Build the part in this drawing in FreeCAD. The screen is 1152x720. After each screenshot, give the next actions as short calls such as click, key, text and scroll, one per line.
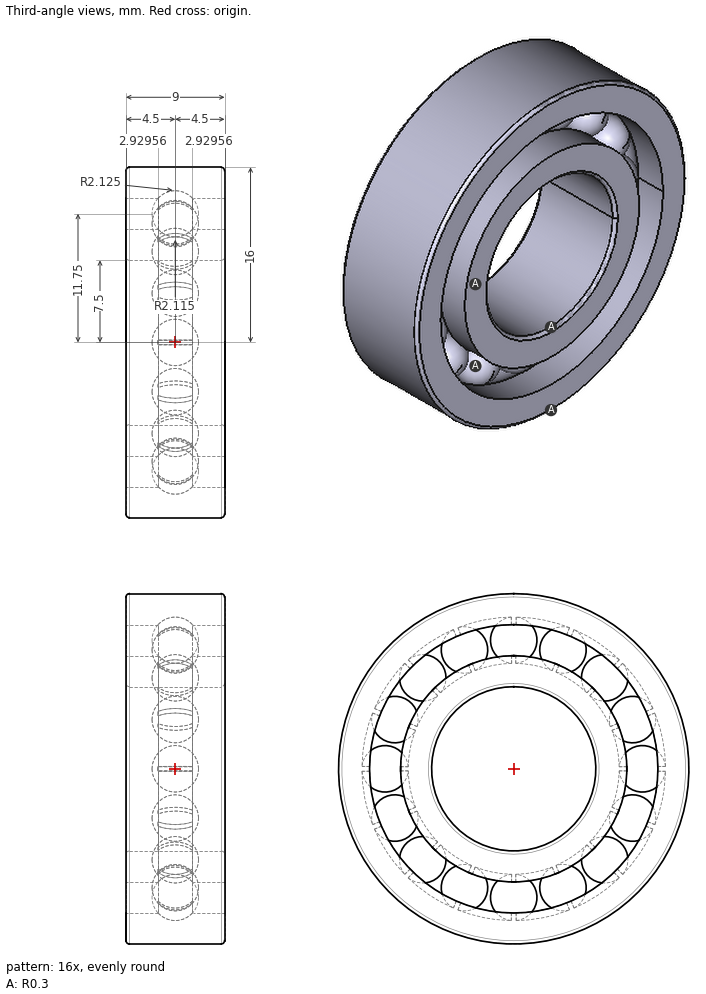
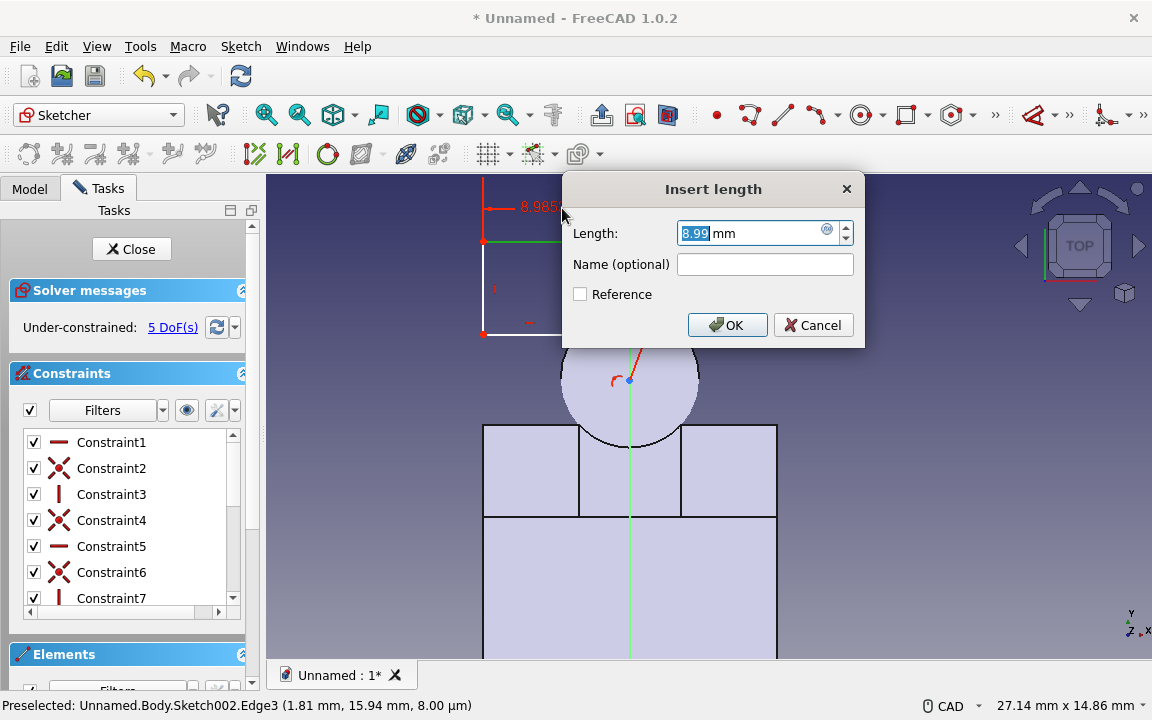
text(9)
key(Return)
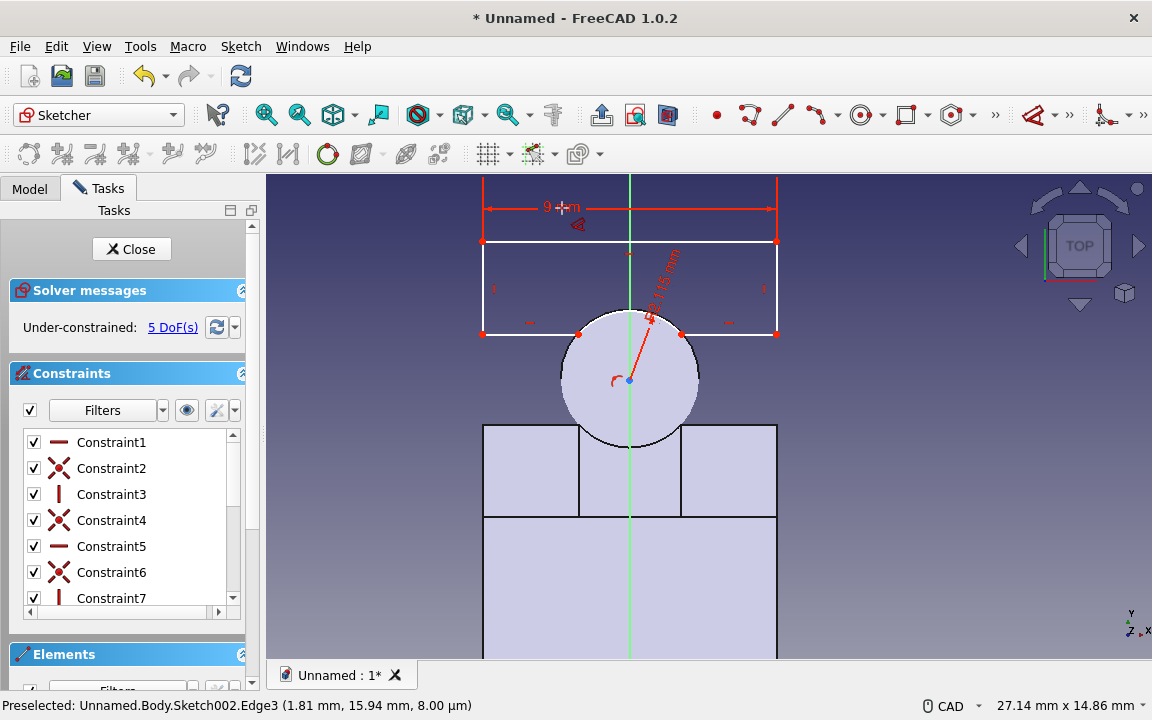
click(777, 242)
click(811, 436)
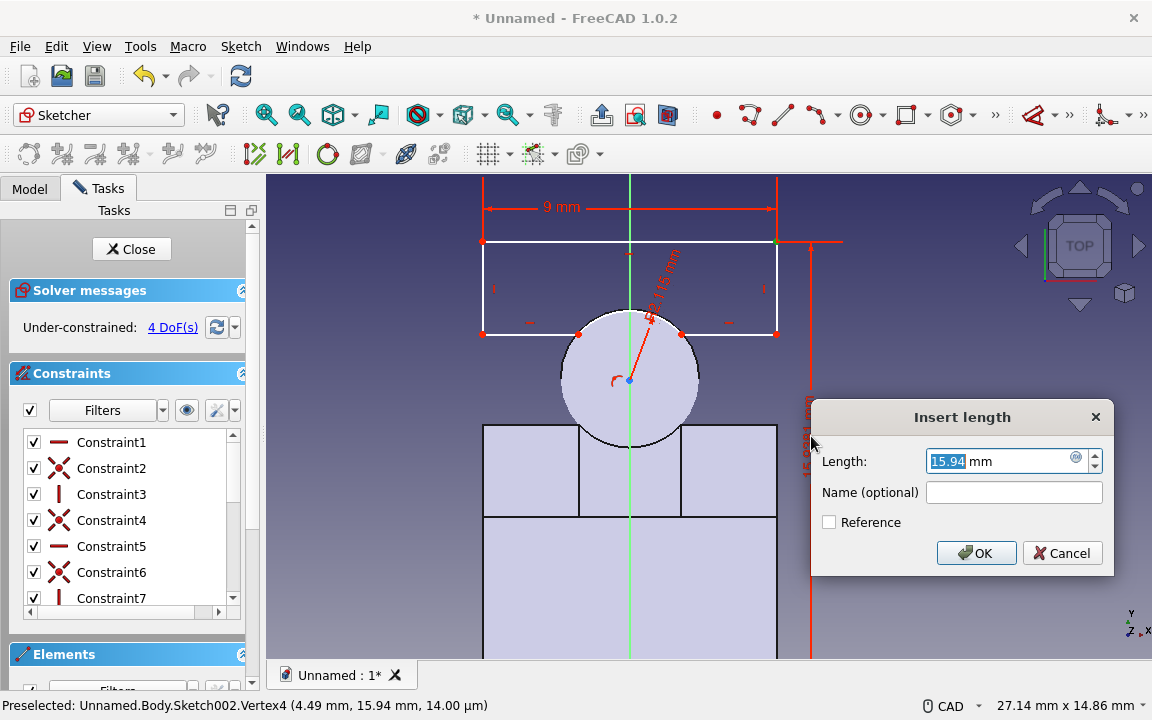
text(16)
key(Return)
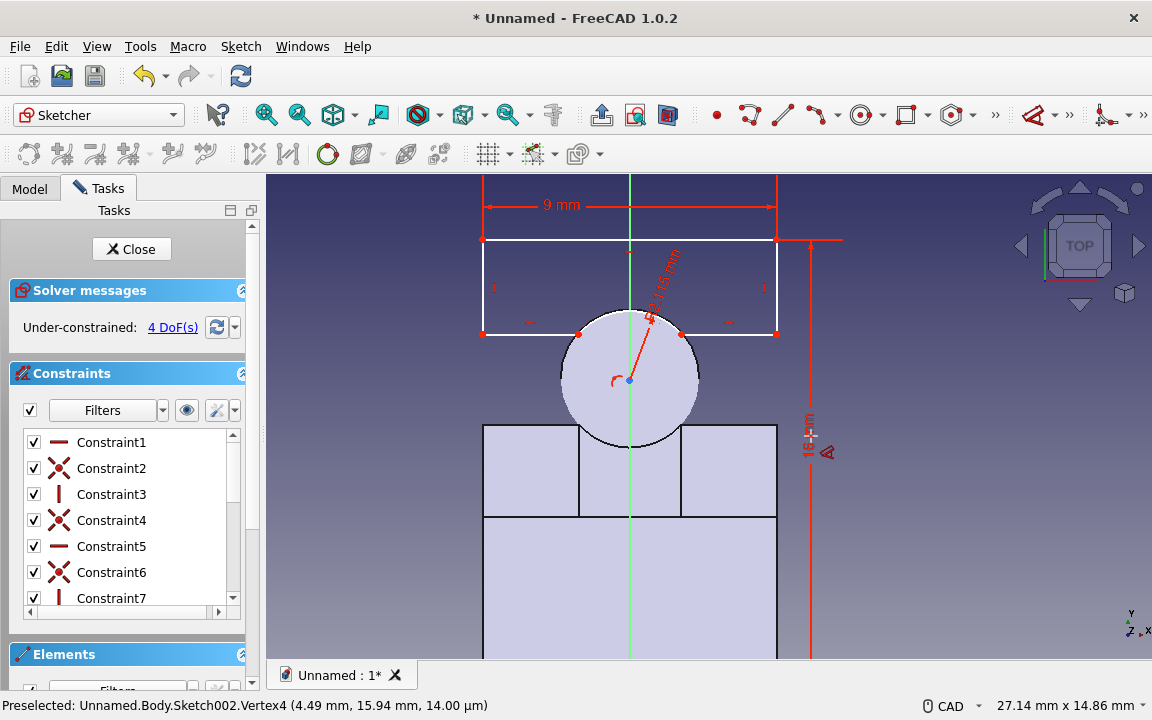
click(777, 335)
click(737, 301)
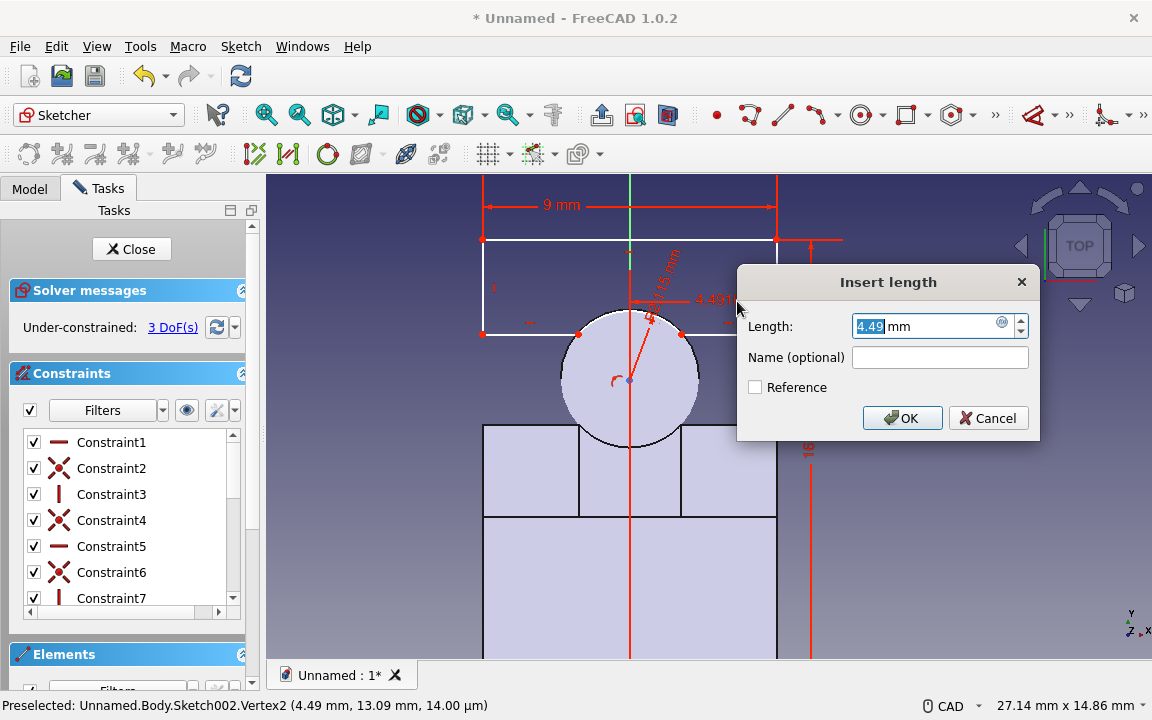
text(4.5)
key(Return)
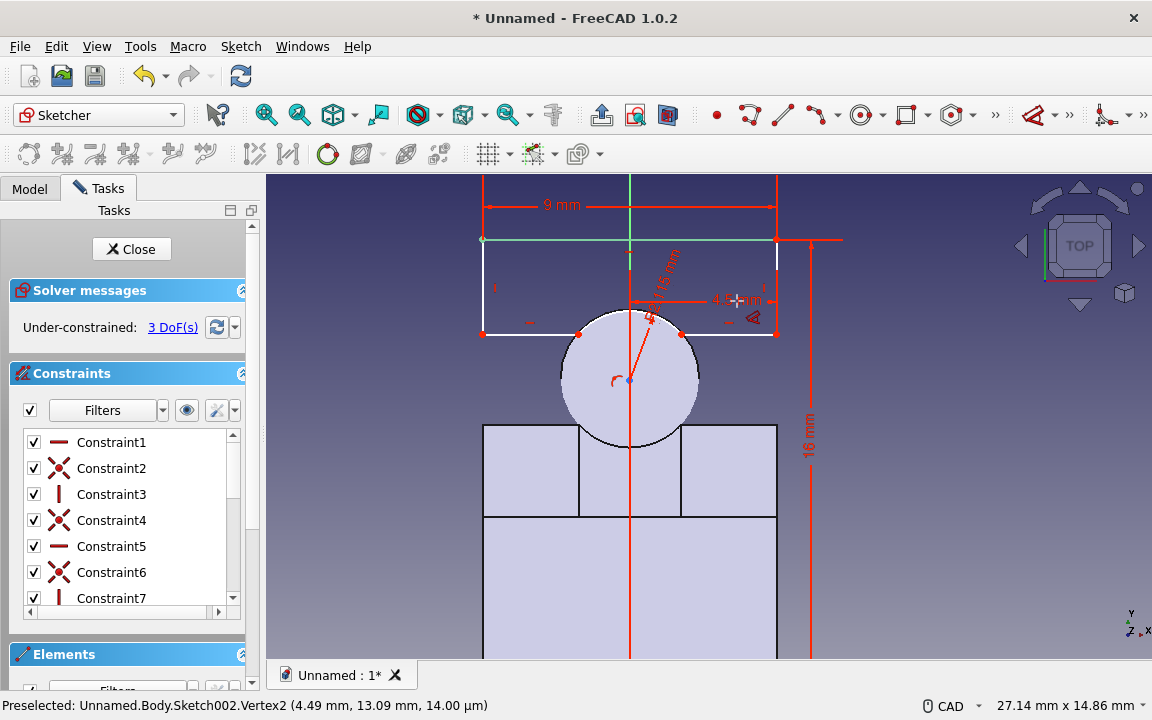
click(630, 380)
click(664, 506)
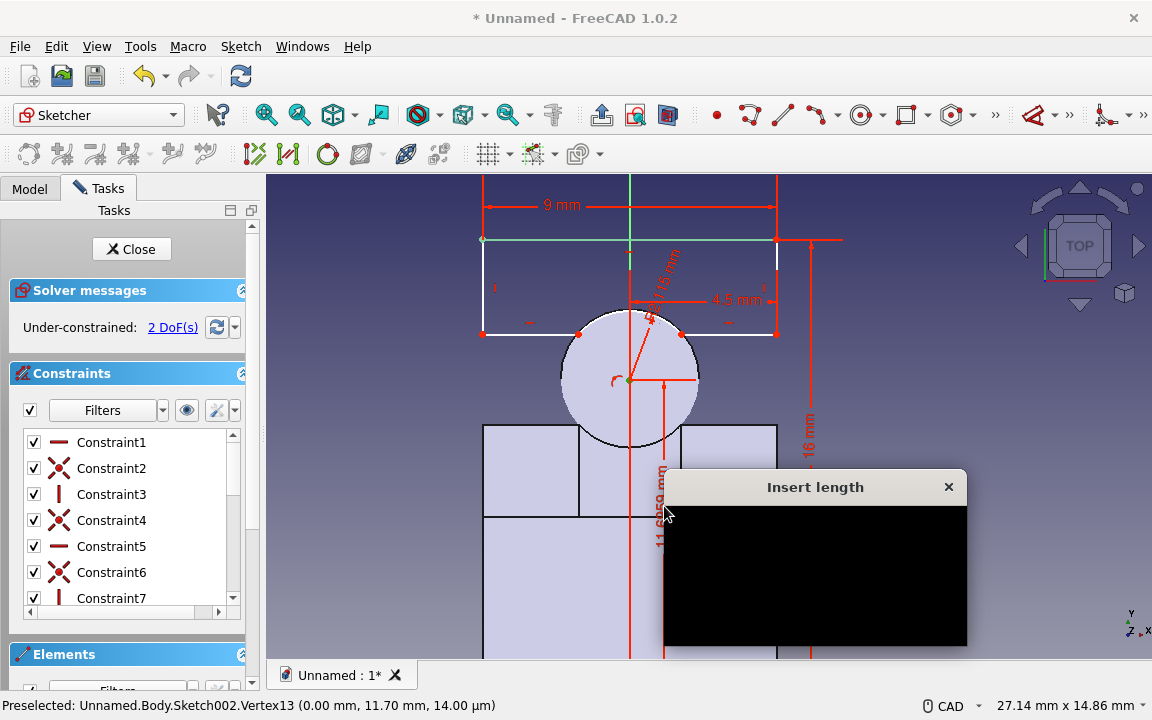
text(11.75)
key(Return)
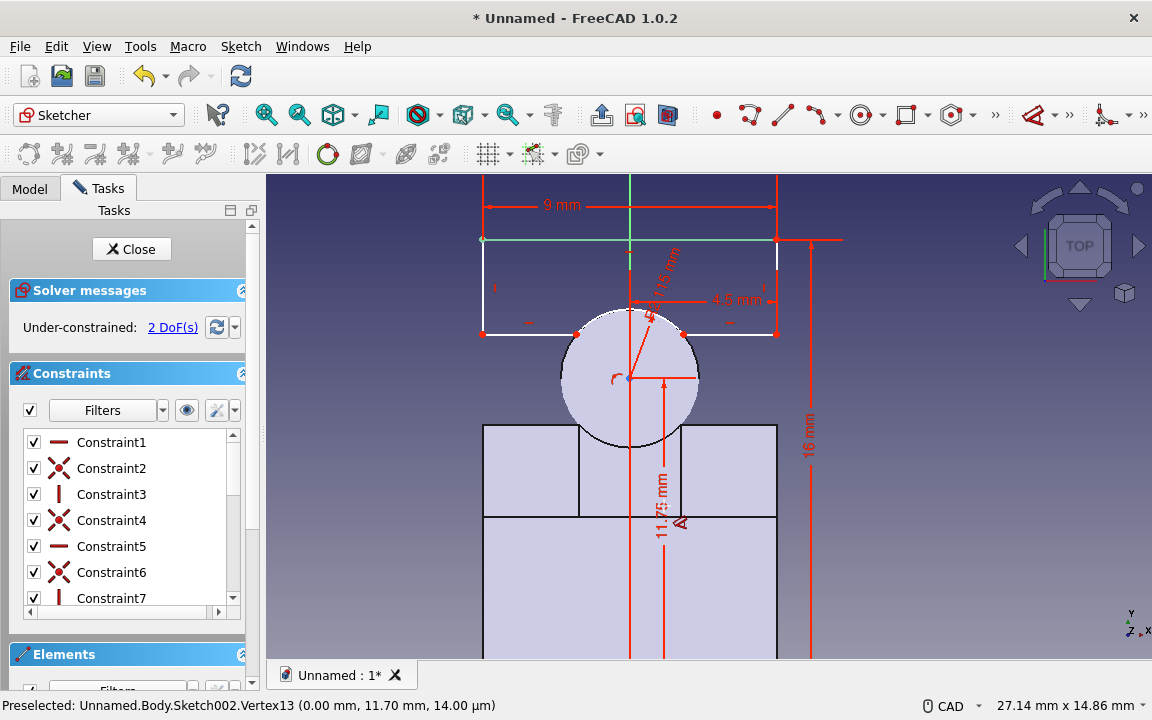
click(711, 335)
click(730, 369)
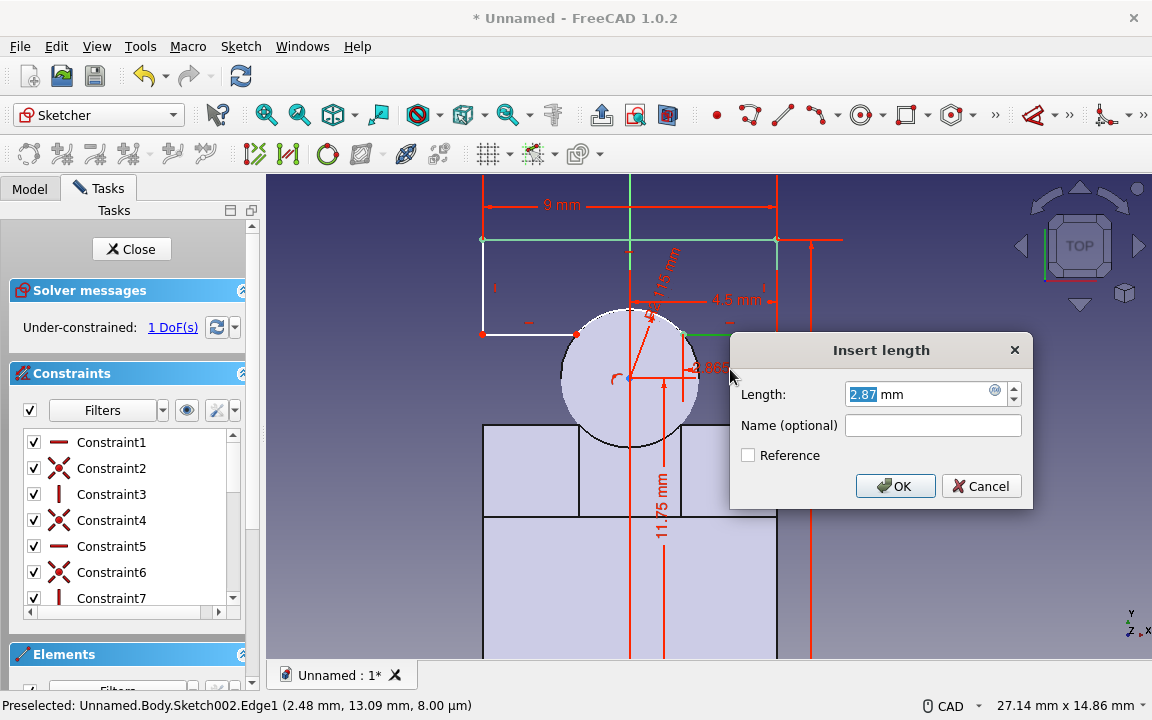
text(2.92956)
key(Return)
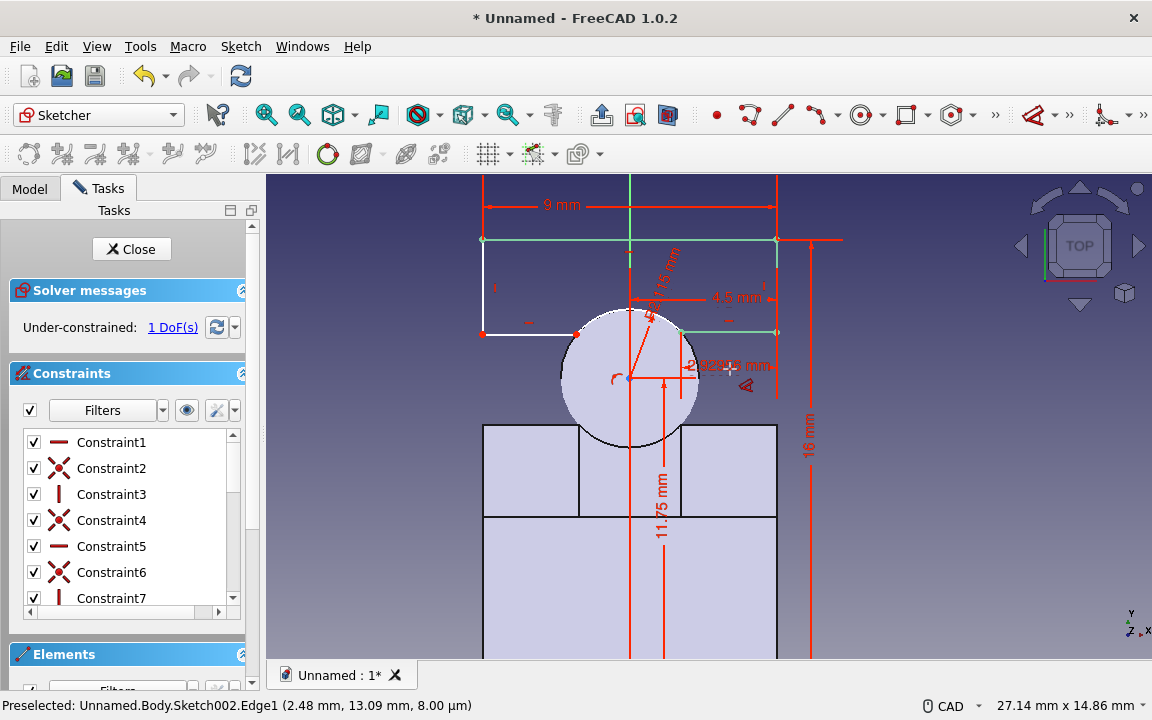
click(511, 335)
click(530, 301)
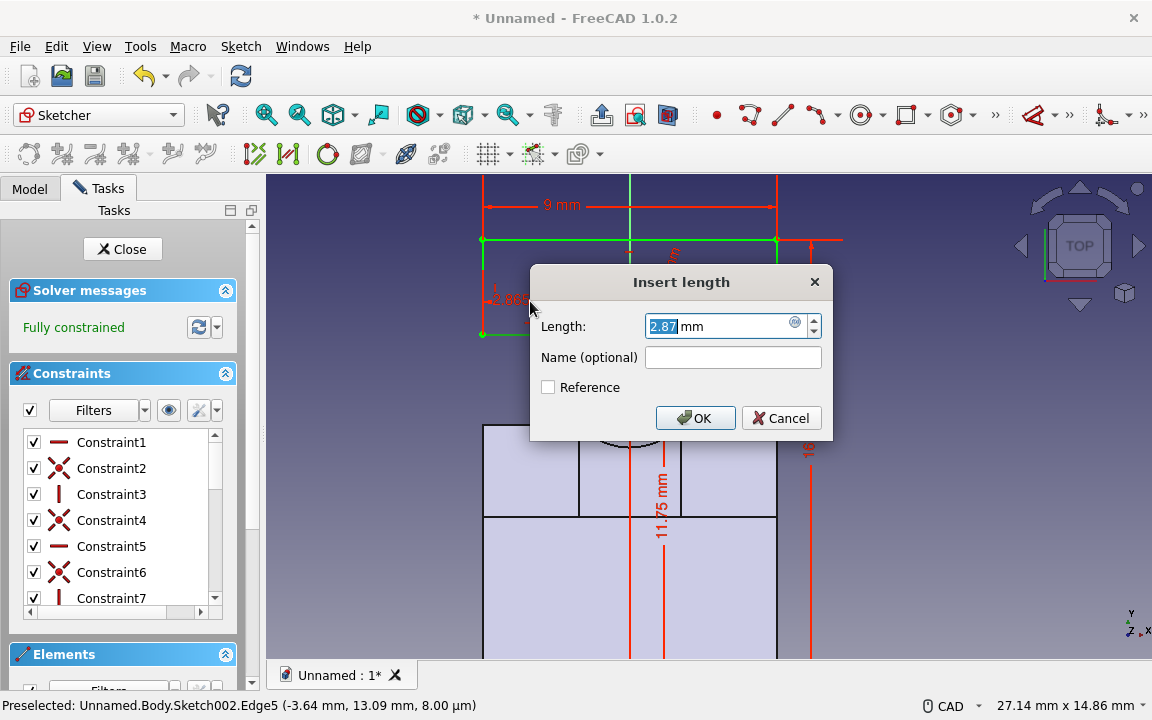
text(2.92956)
key(Return)
key(Escape)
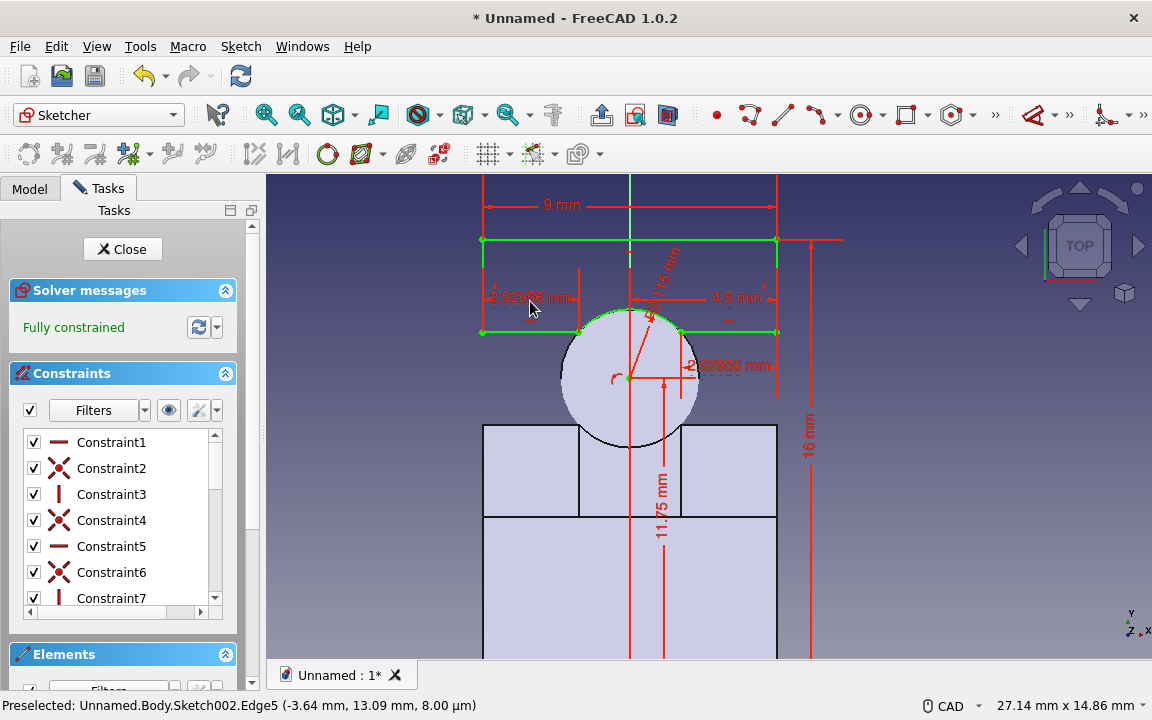
click(123, 249)